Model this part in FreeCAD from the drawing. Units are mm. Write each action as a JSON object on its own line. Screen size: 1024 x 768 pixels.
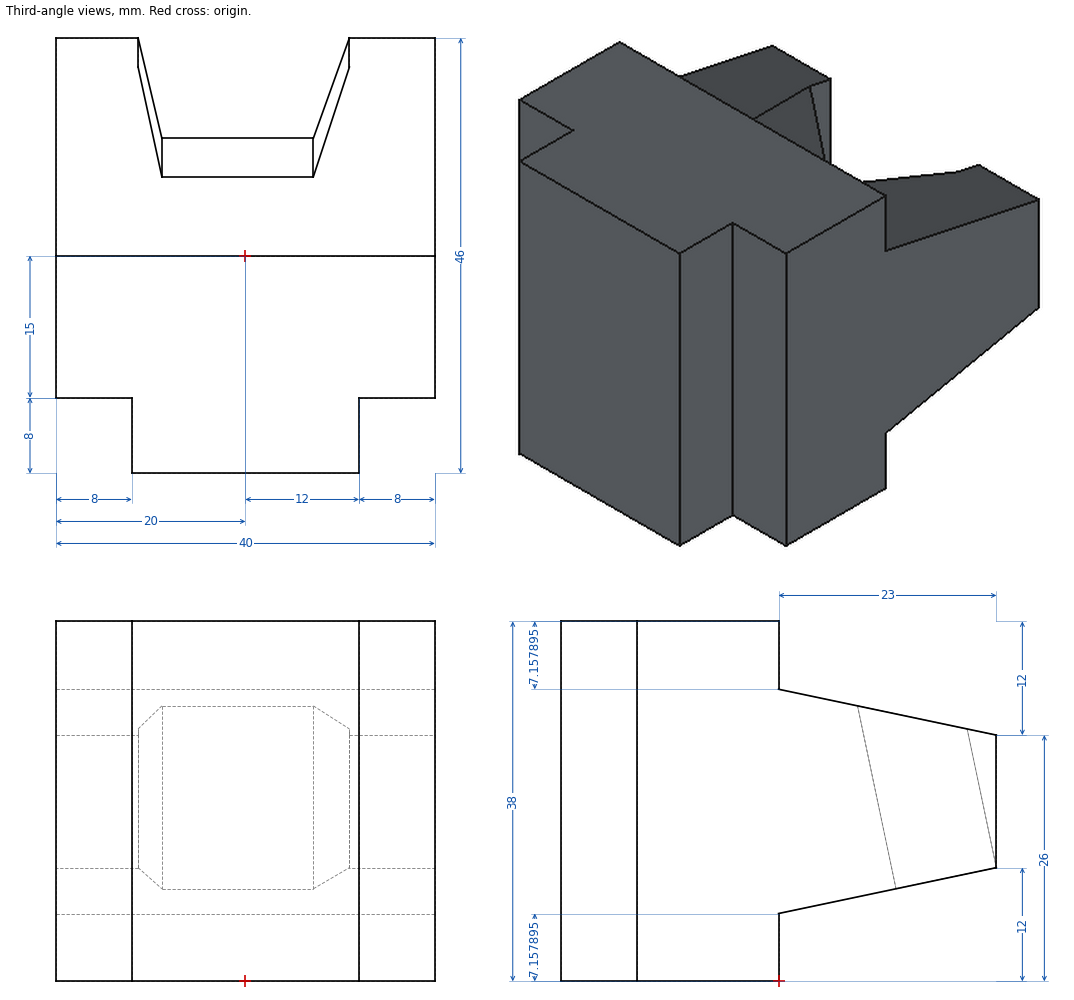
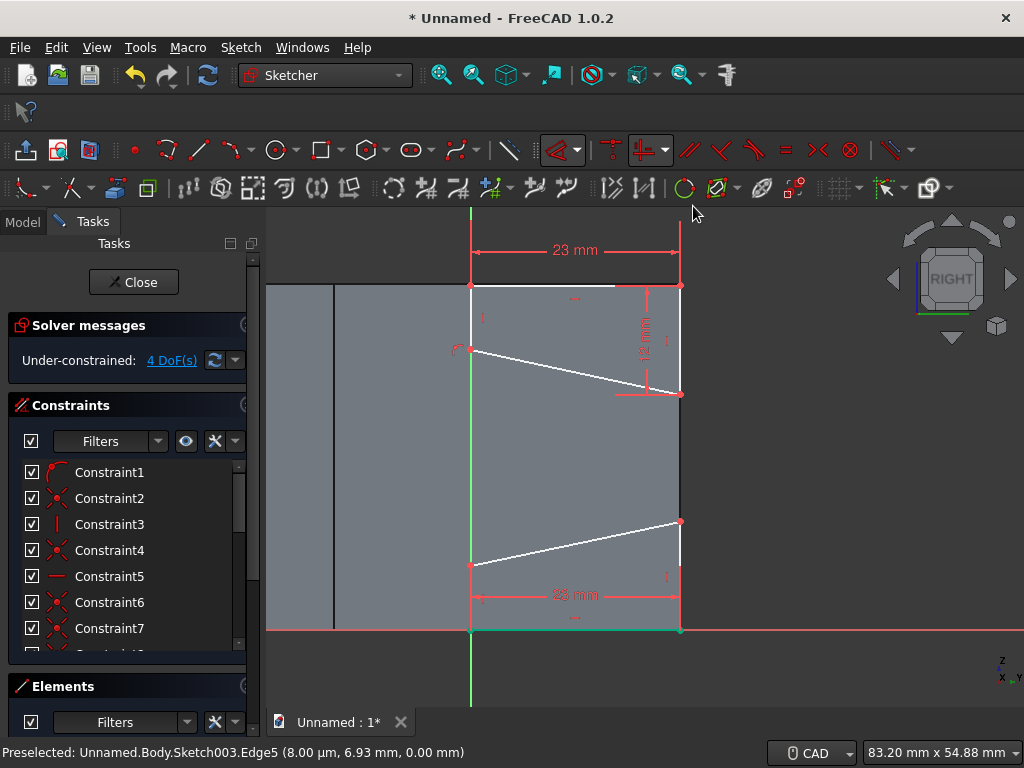
{"action": "left_click", "coordinate": [680, 598]}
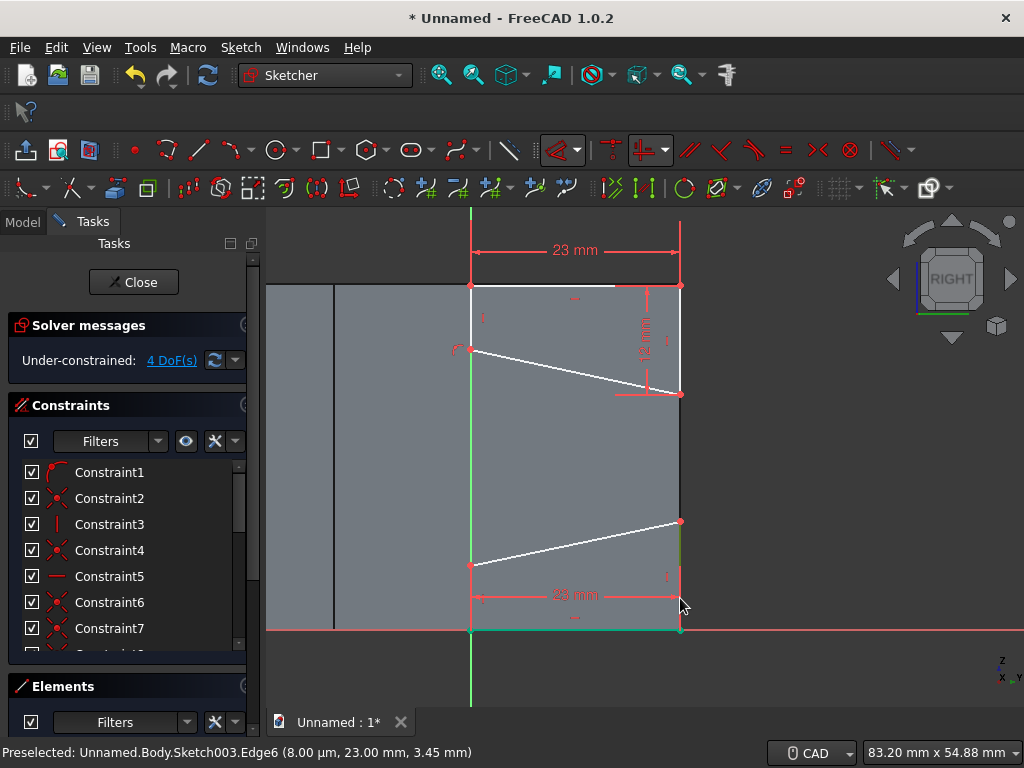
{"action": "key", "text": "i"}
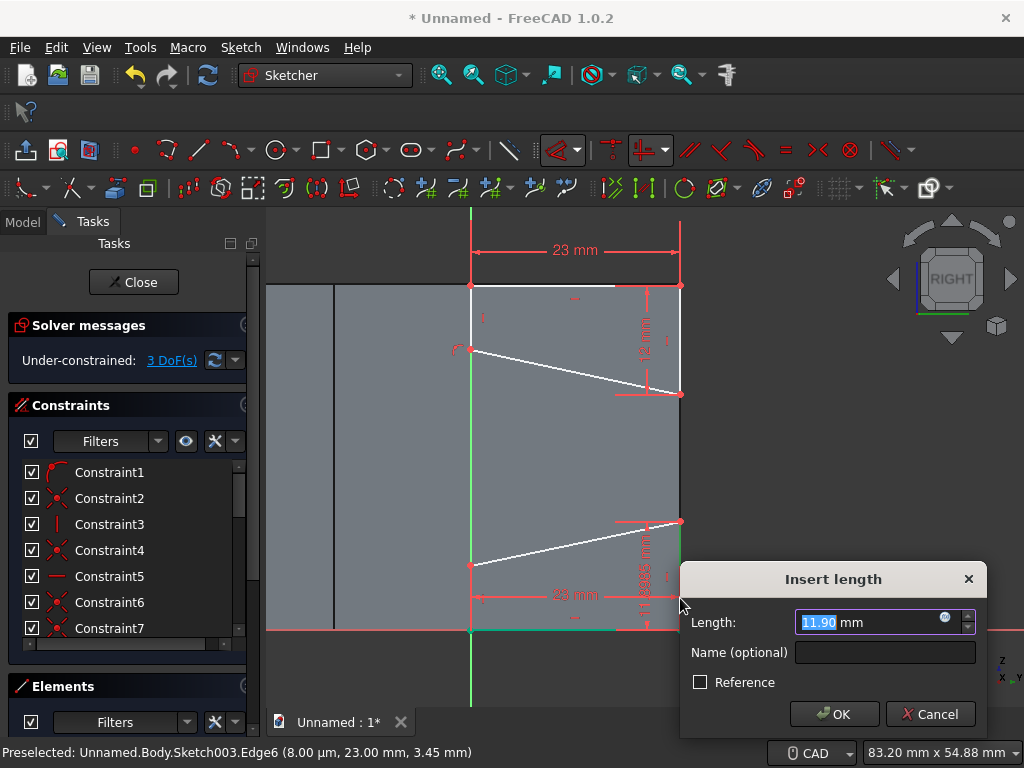
{"action": "type", "text": "12"}
{"action": "key", "text": "Return"}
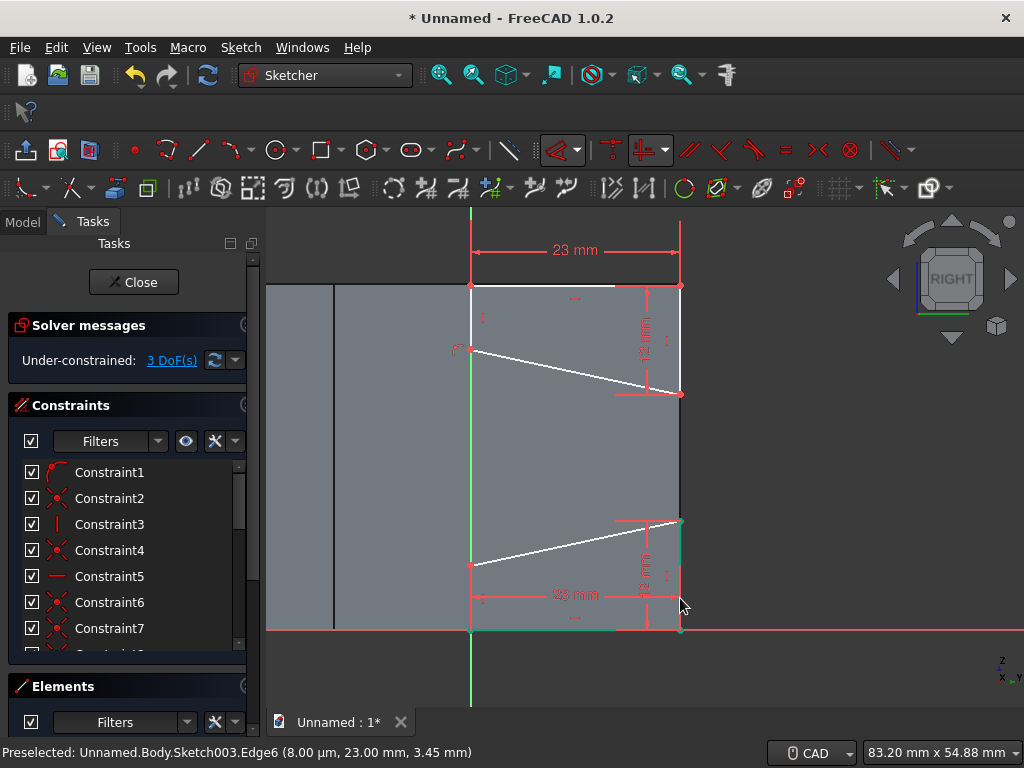
{"action": "left_click", "coordinate": [680, 395]}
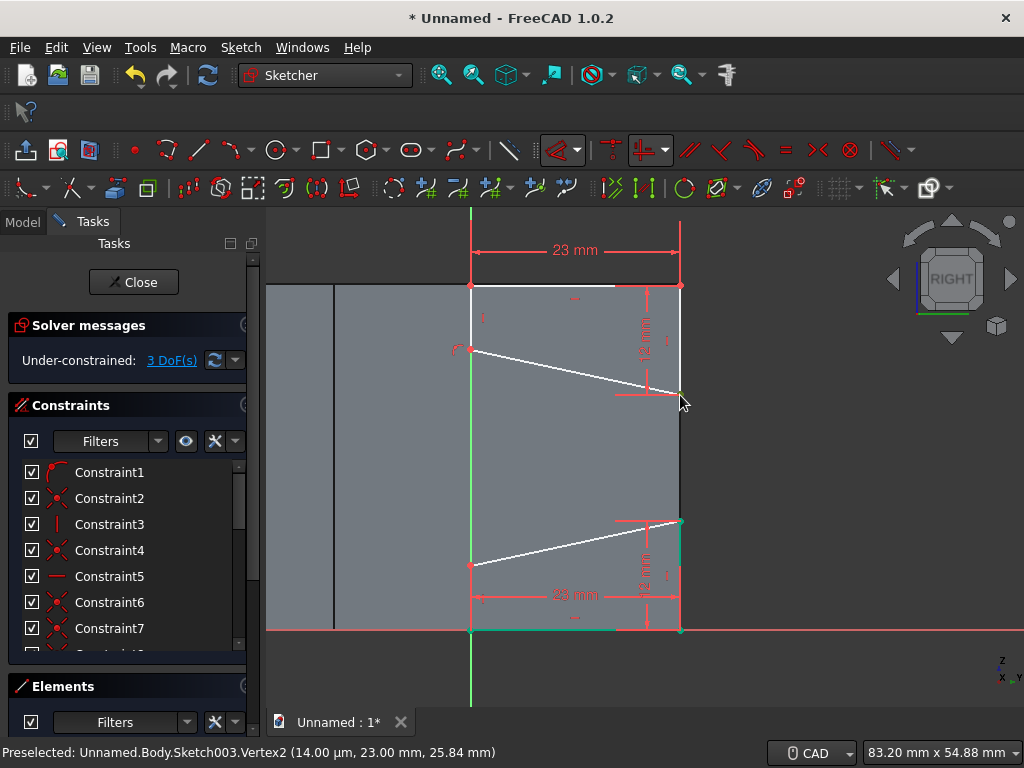
{"action": "key", "text": "i"}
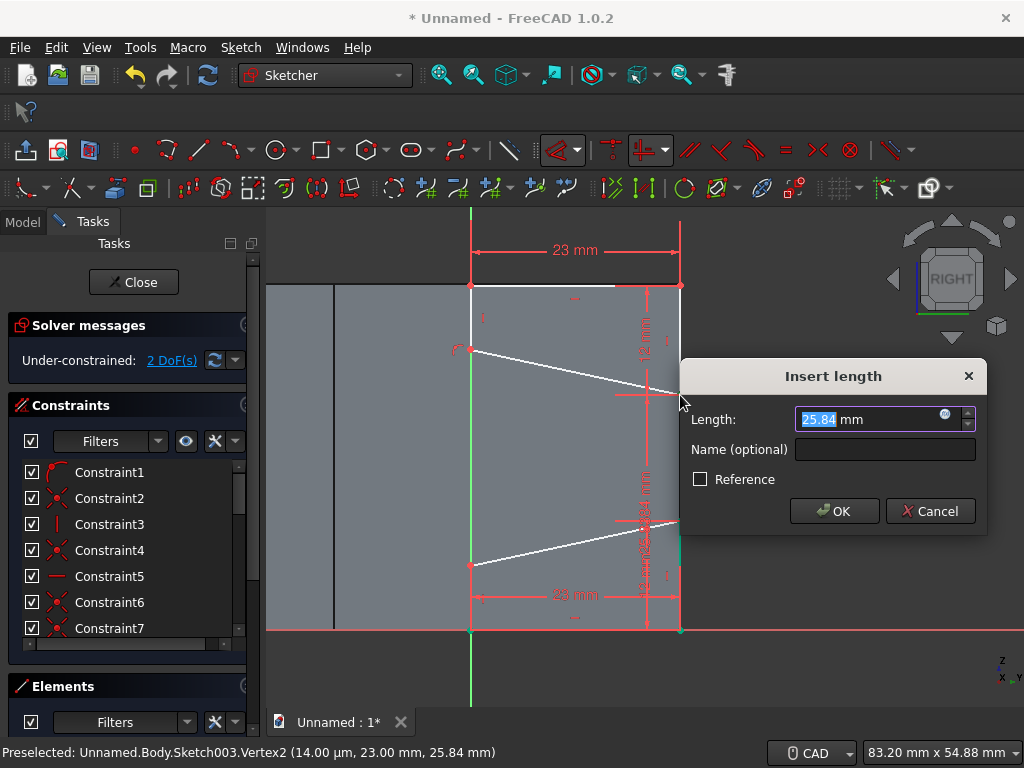
{"action": "type", "text": "26"}
{"action": "key", "text": "Return"}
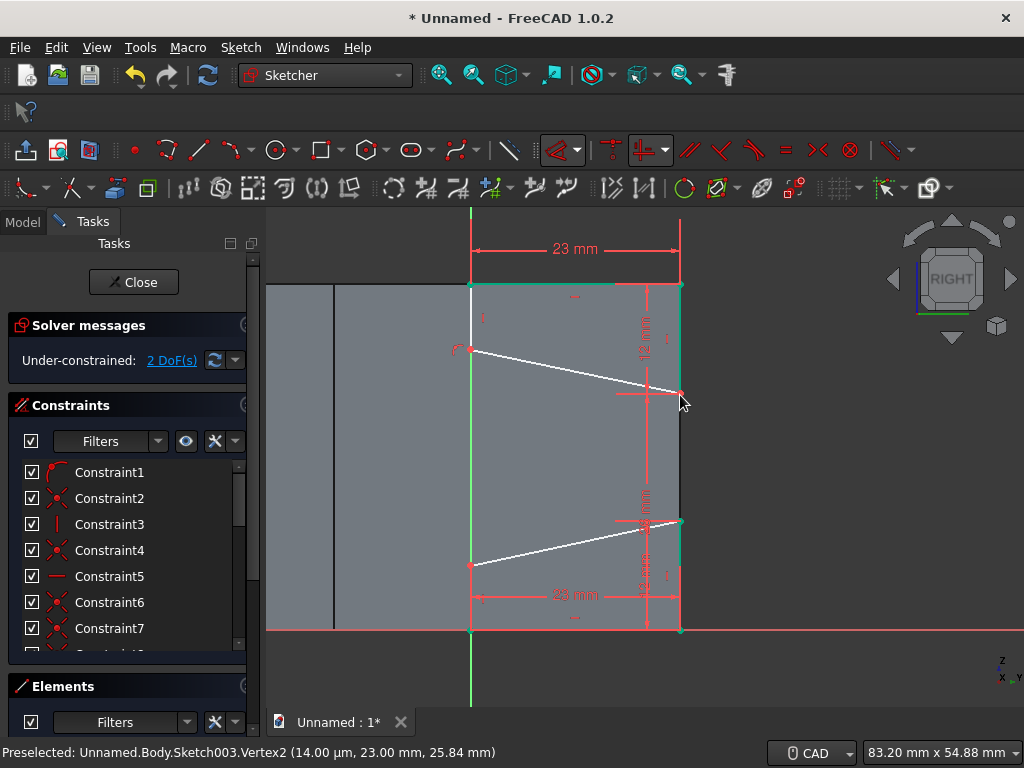
{"action": "left_click", "coordinate": [471, 304]}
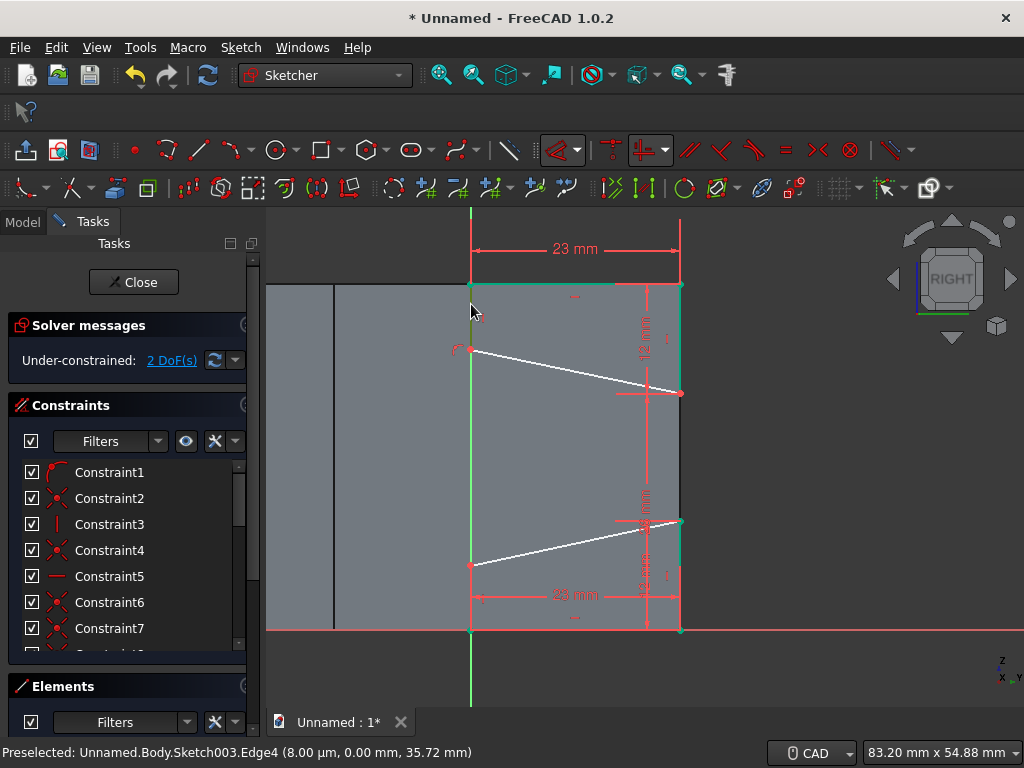
{"action": "left_click", "coordinate": [580, 150]}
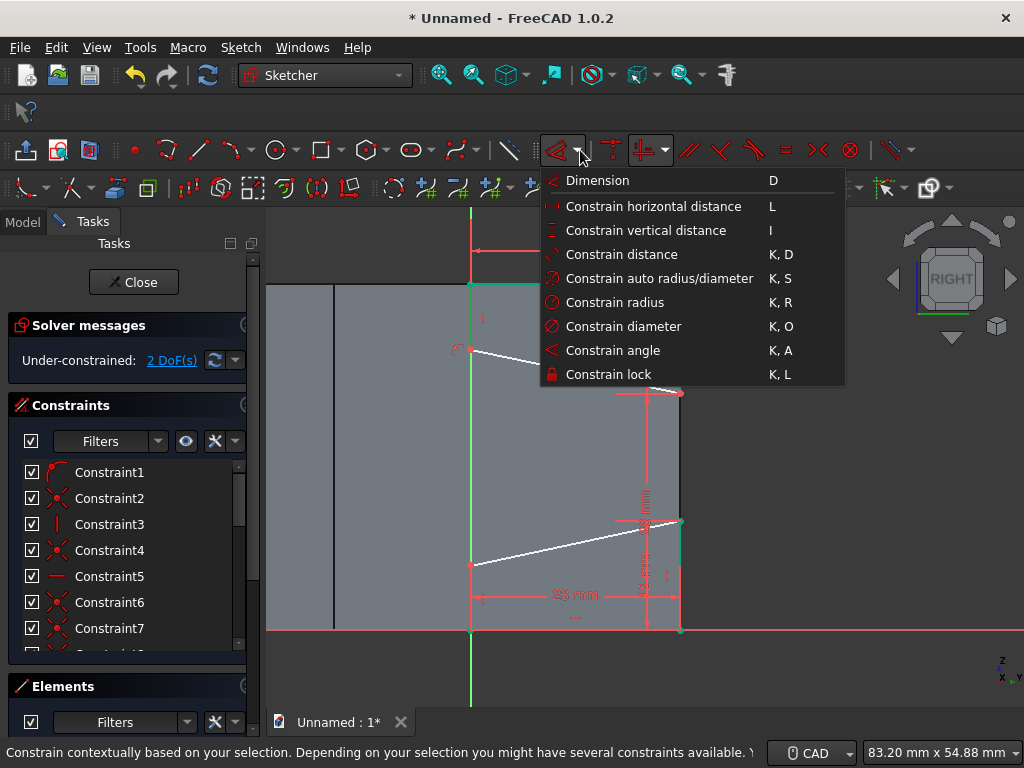
{"action": "left_click", "coordinate": [693, 230]}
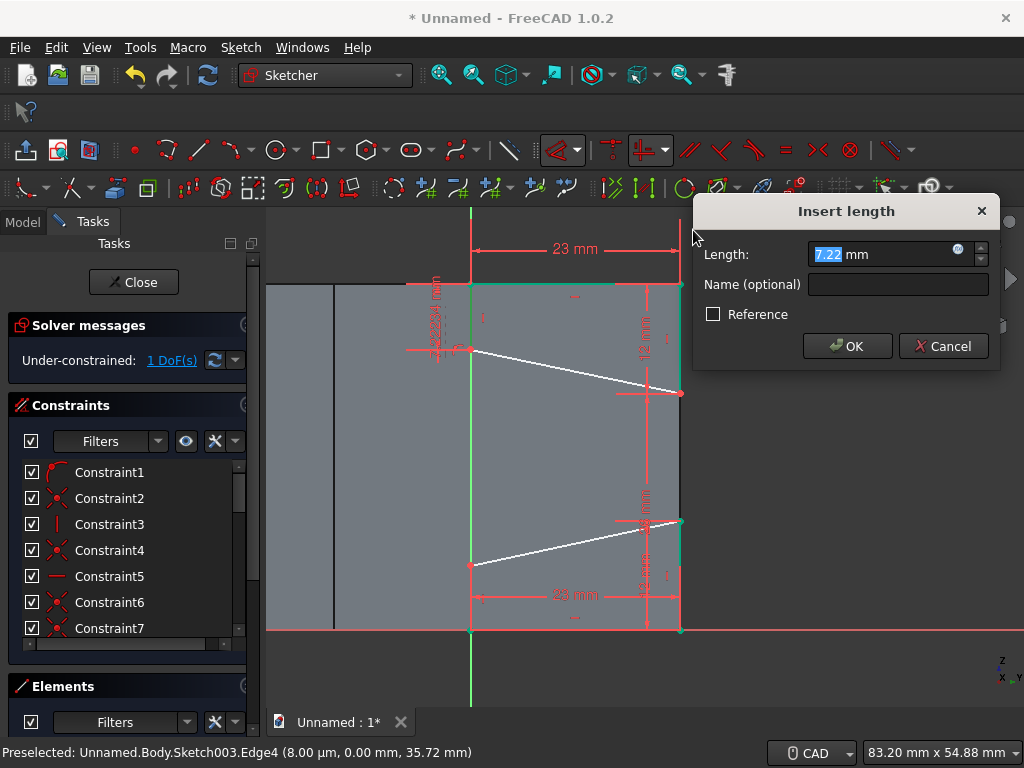
{"action": "type", "text": "7.157895"}
{"action": "key", "text": "Return"}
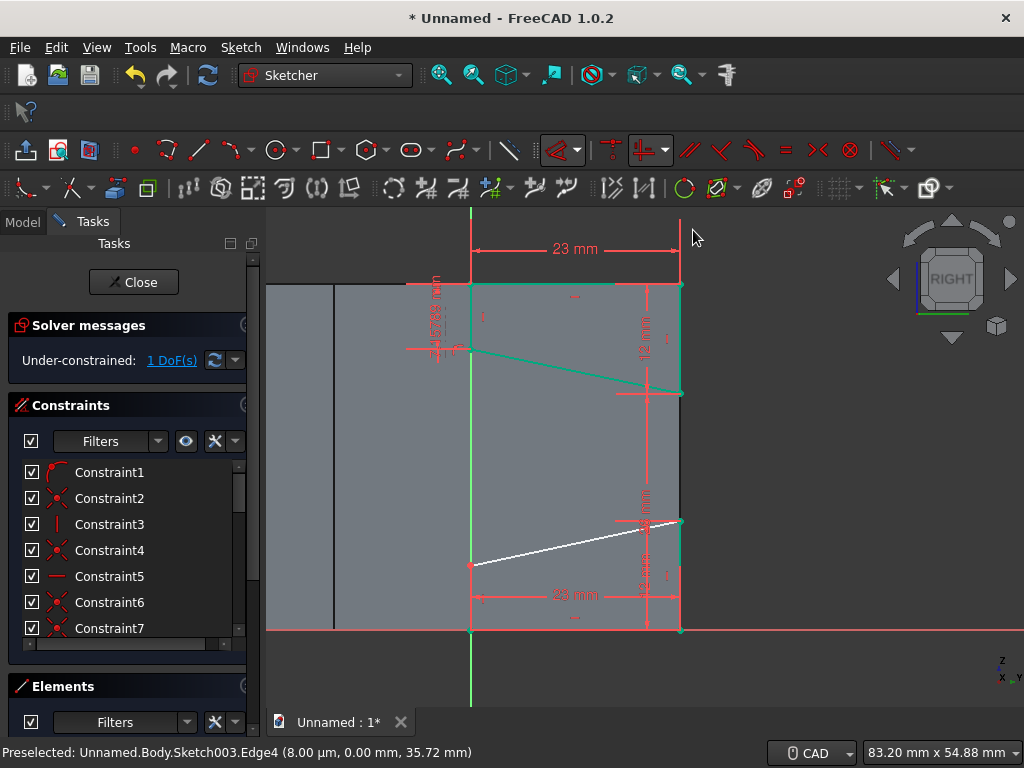
{"action": "left_click", "coordinate": [471, 585]}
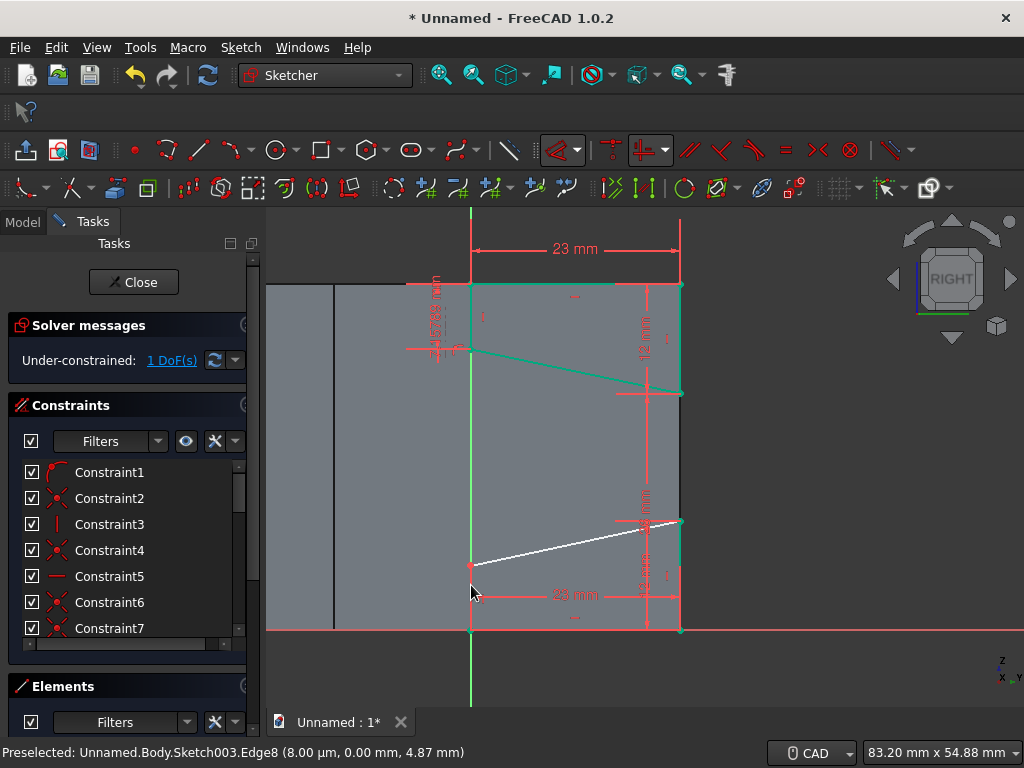
{"action": "key", "text": "i"}